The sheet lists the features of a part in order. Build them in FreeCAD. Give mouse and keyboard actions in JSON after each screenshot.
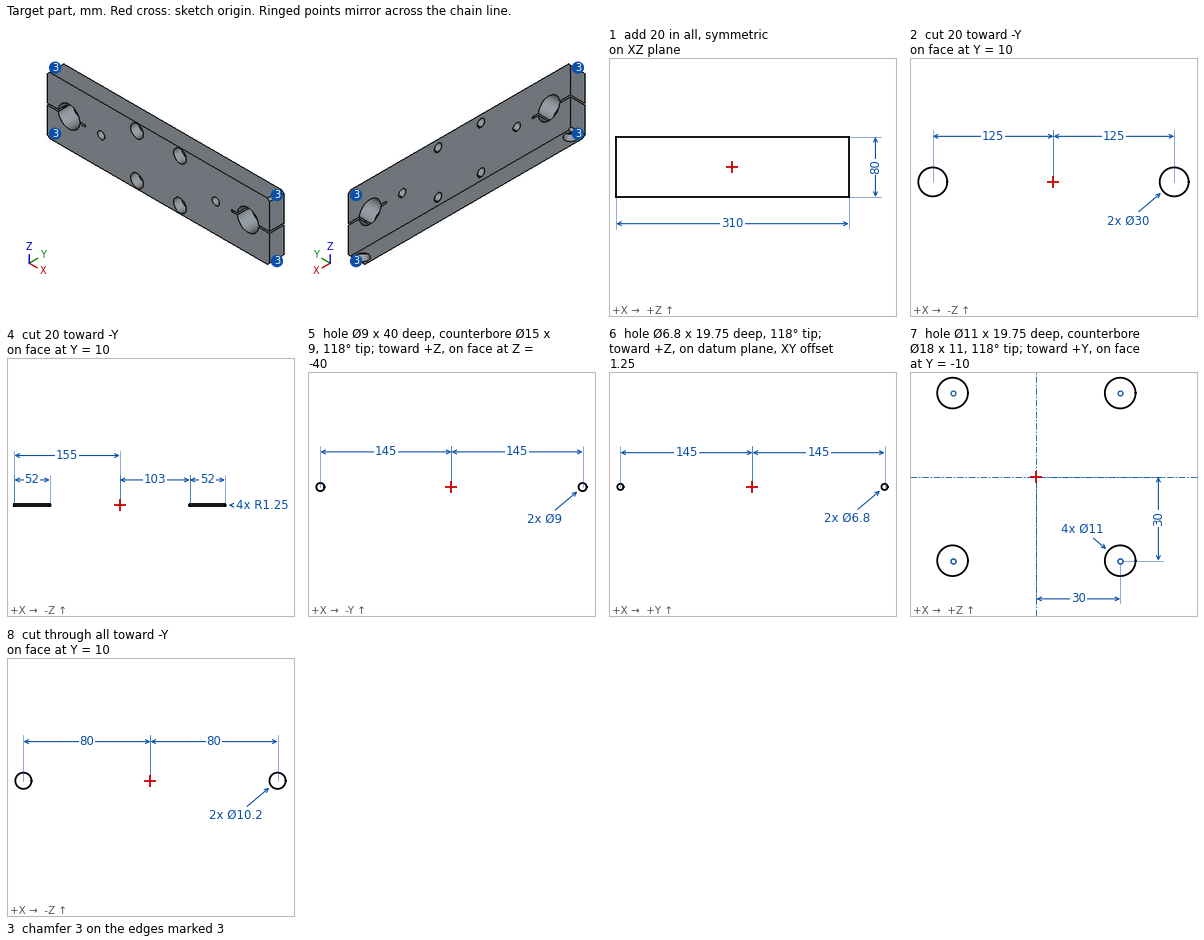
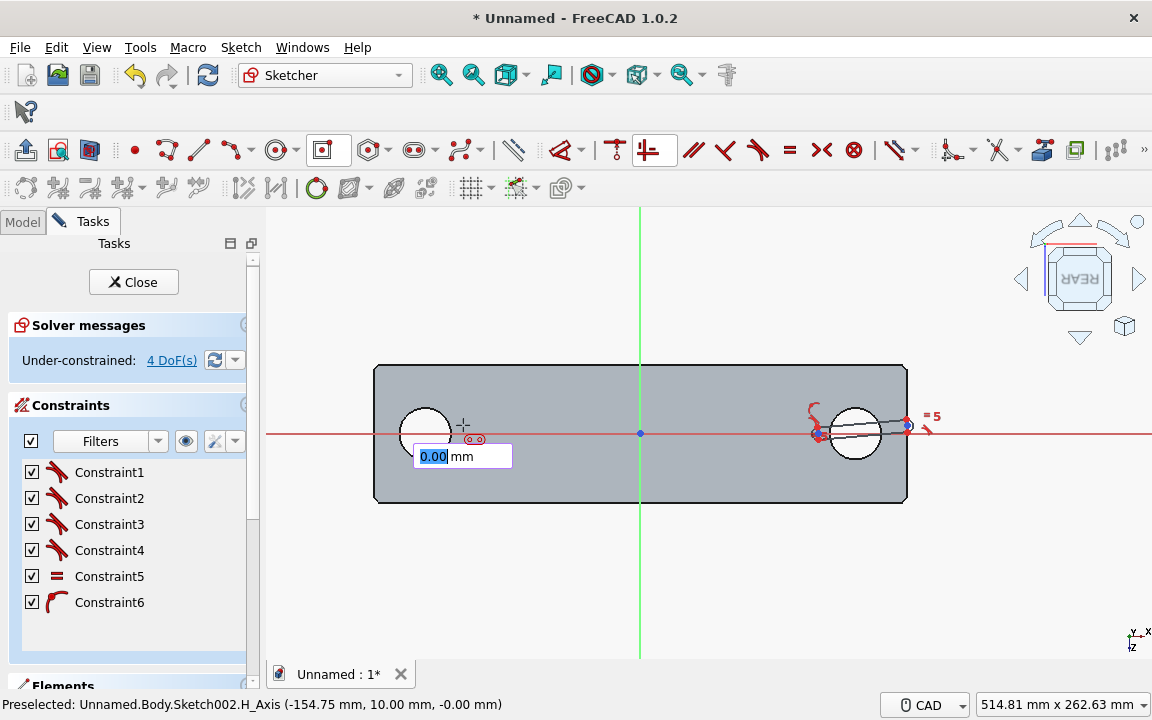
{"action": "scroll", "coordinate": [418, 436], "scroll_direction": "up", "scroll_amount": 10}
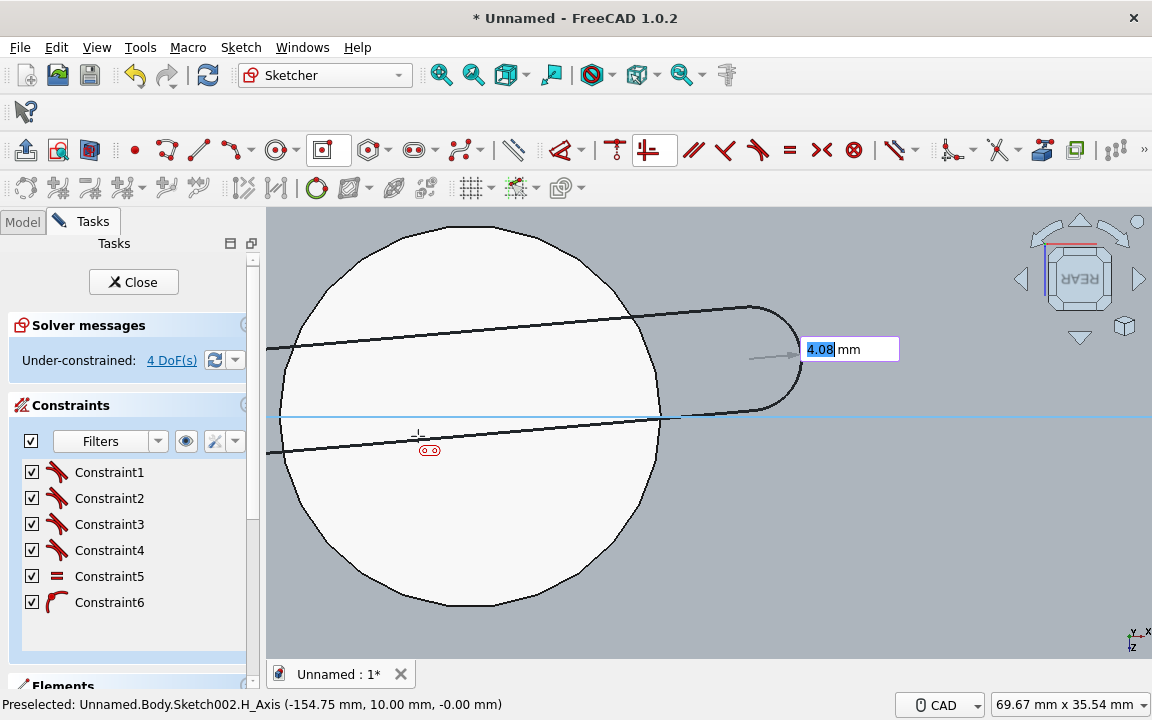
{"action": "left_click", "coordinate": [419, 432]}
{"action": "key", "text": "Escape"}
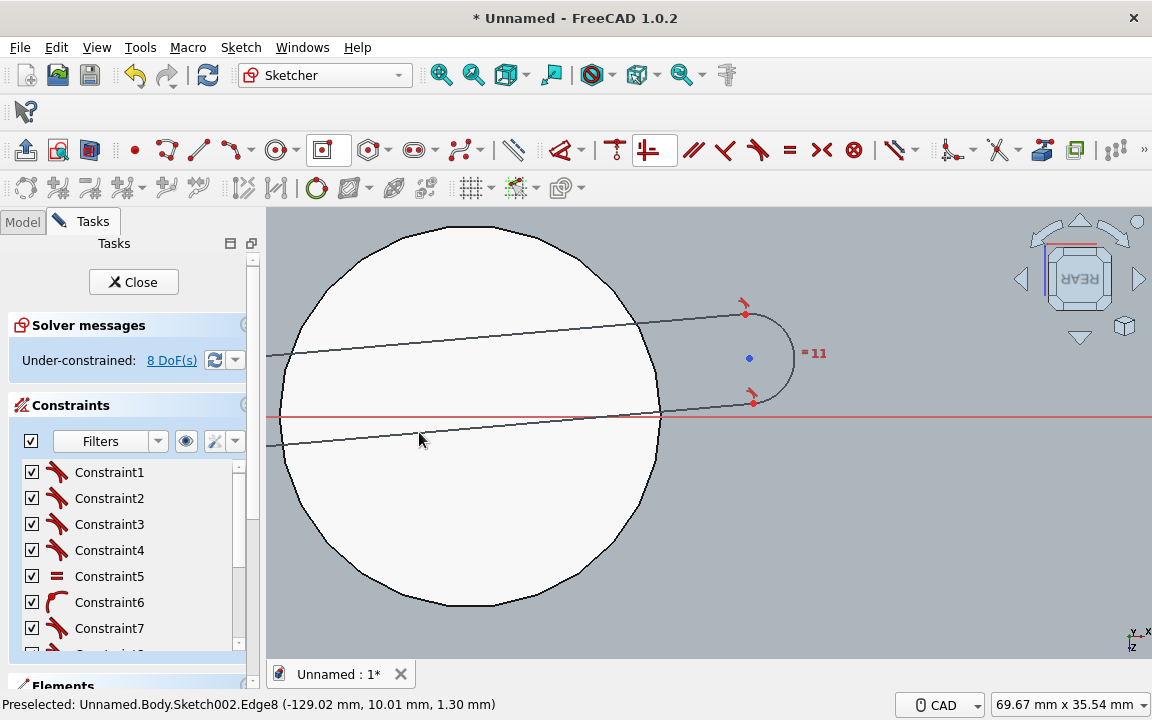
{"action": "scroll", "coordinate": [418, 436], "scroll_direction": "down", "scroll_amount": 10}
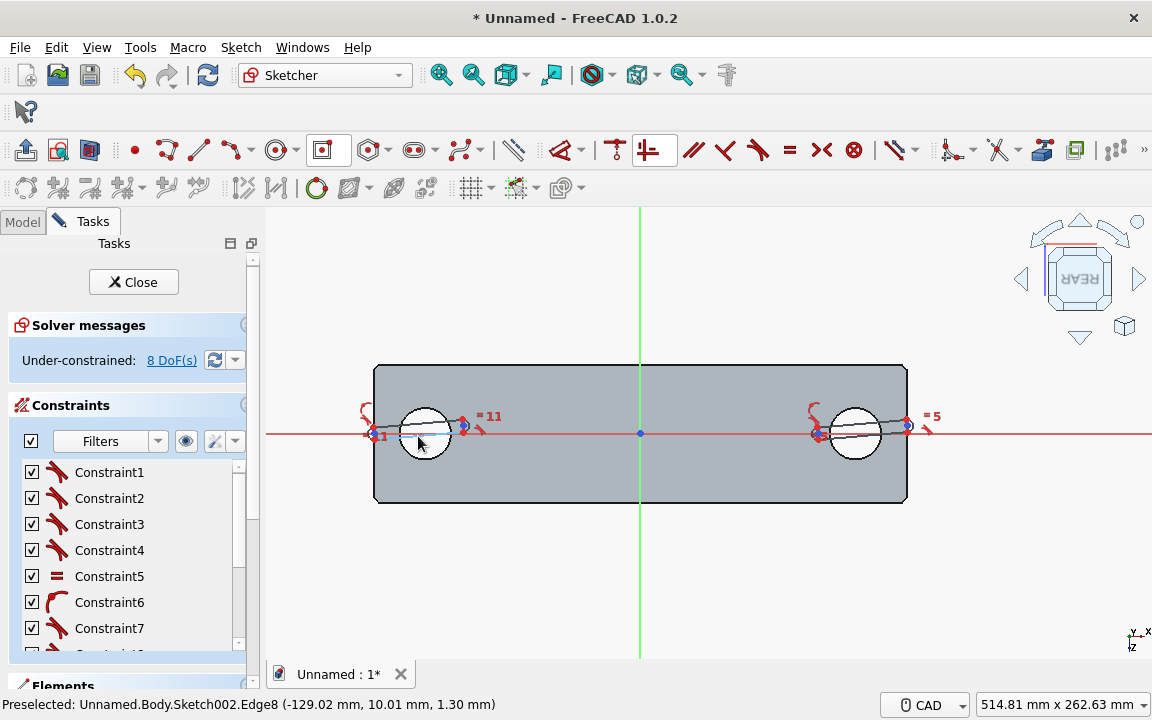
{"action": "scroll", "coordinate": [844, 425], "scroll_direction": "up", "scroll_amount": 3}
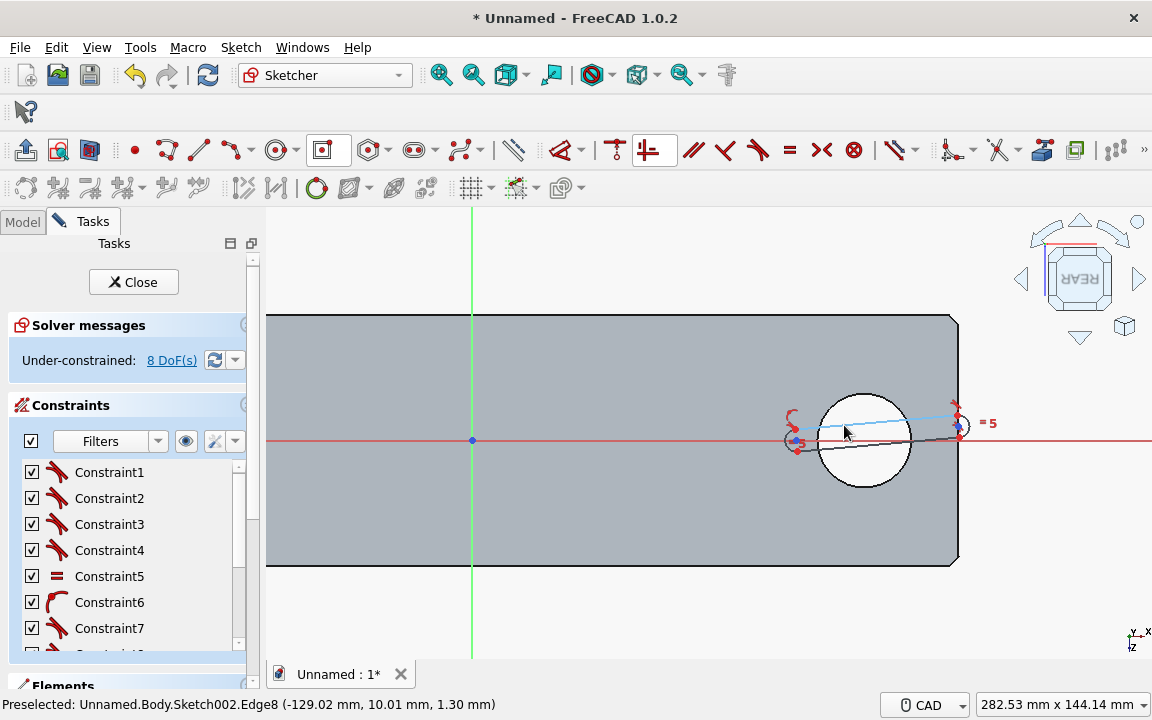
{"action": "left_click", "coordinate": [844, 425]}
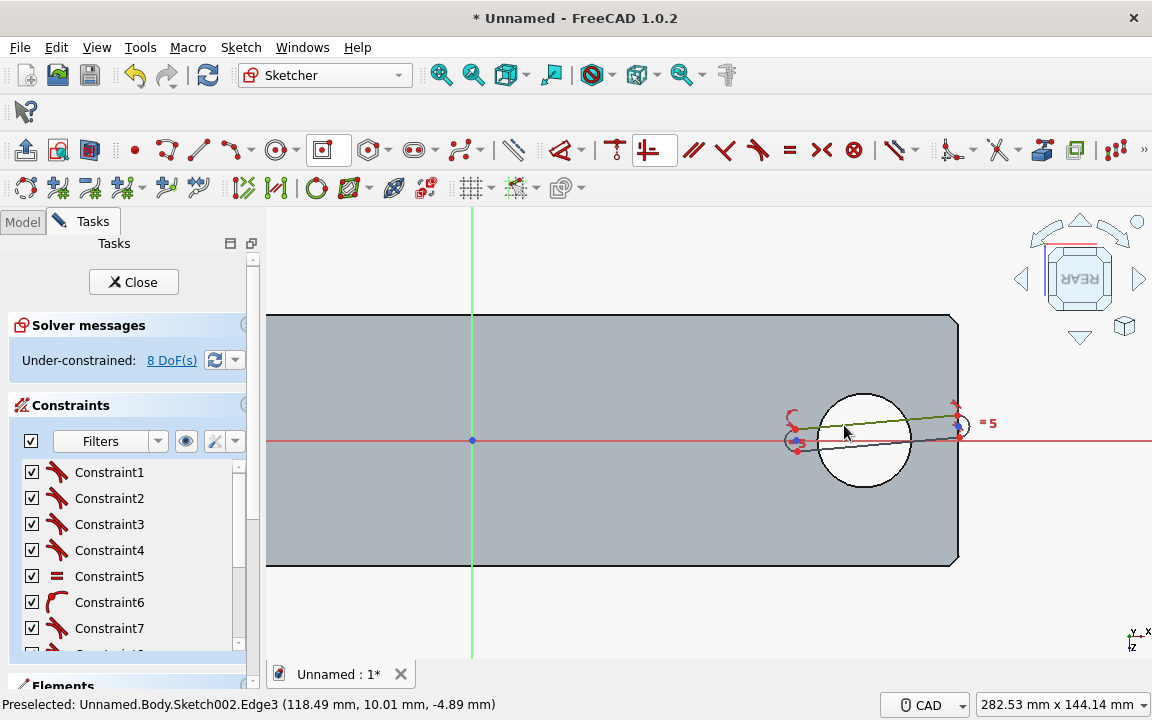
{"action": "key", "text": "h"}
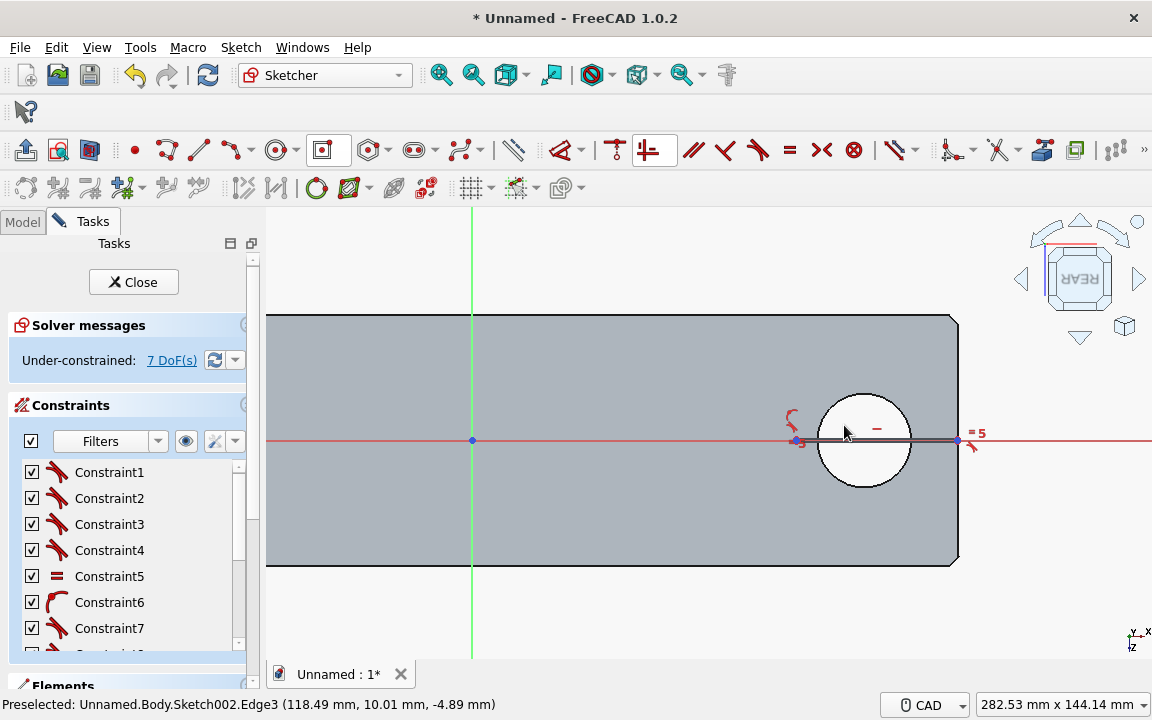
{"action": "scroll", "coordinate": [845, 424], "scroll_direction": "down", "scroll_amount": 3}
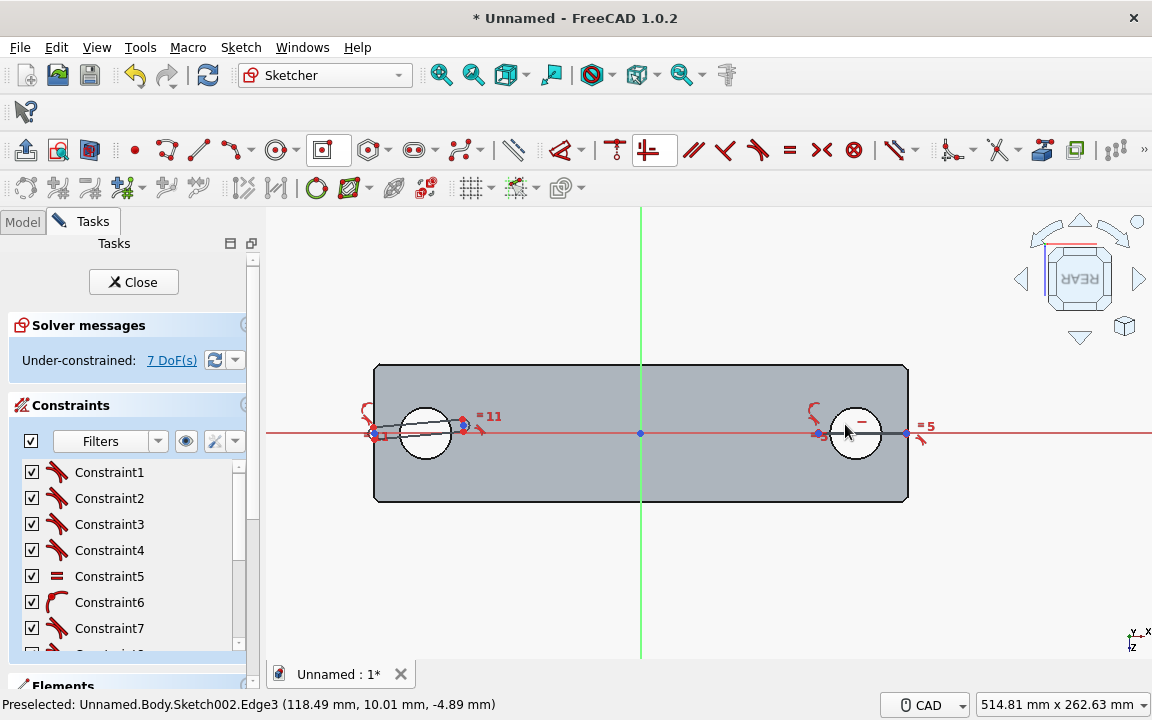
{"action": "scroll", "coordinate": [401, 425], "scroll_direction": "up", "scroll_amount": 3}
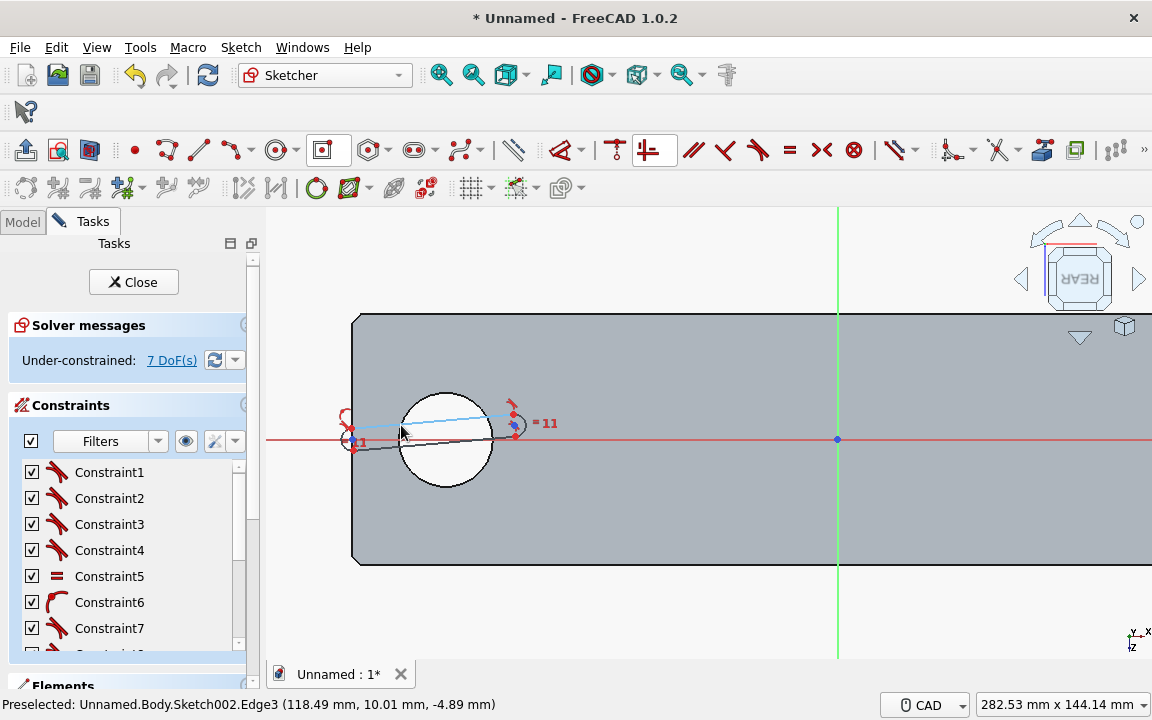
{"action": "left_click", "coordinate": [400, 424]}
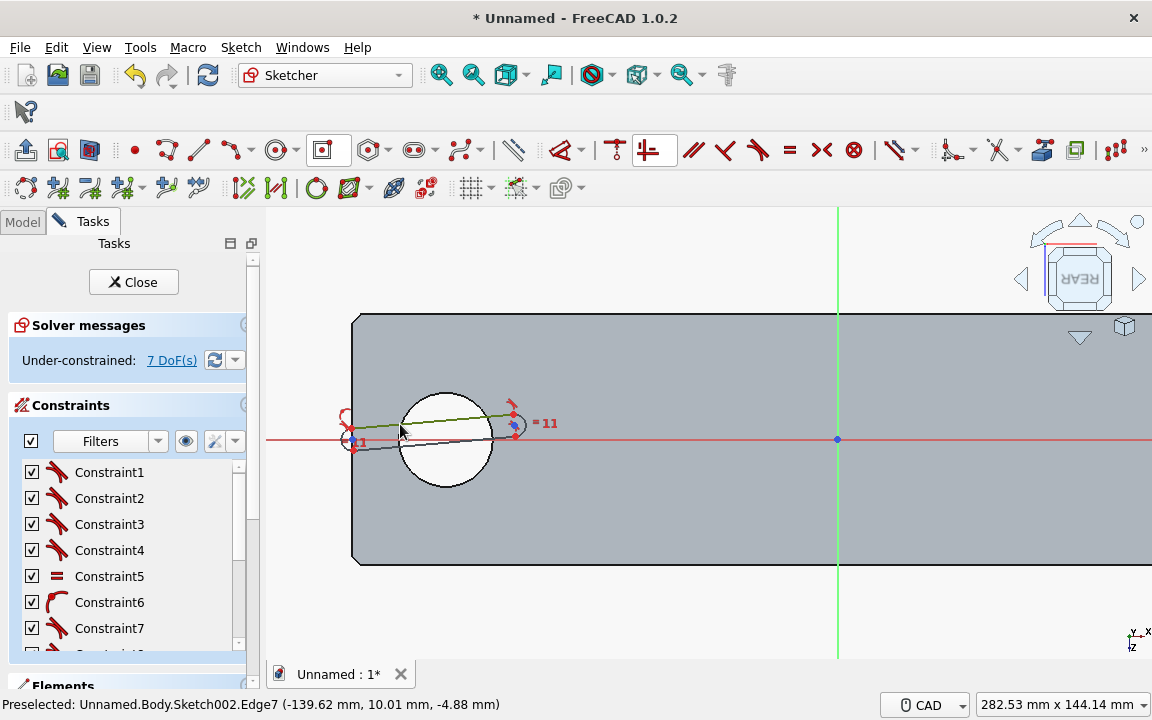
{"action": "key", "text": "h"}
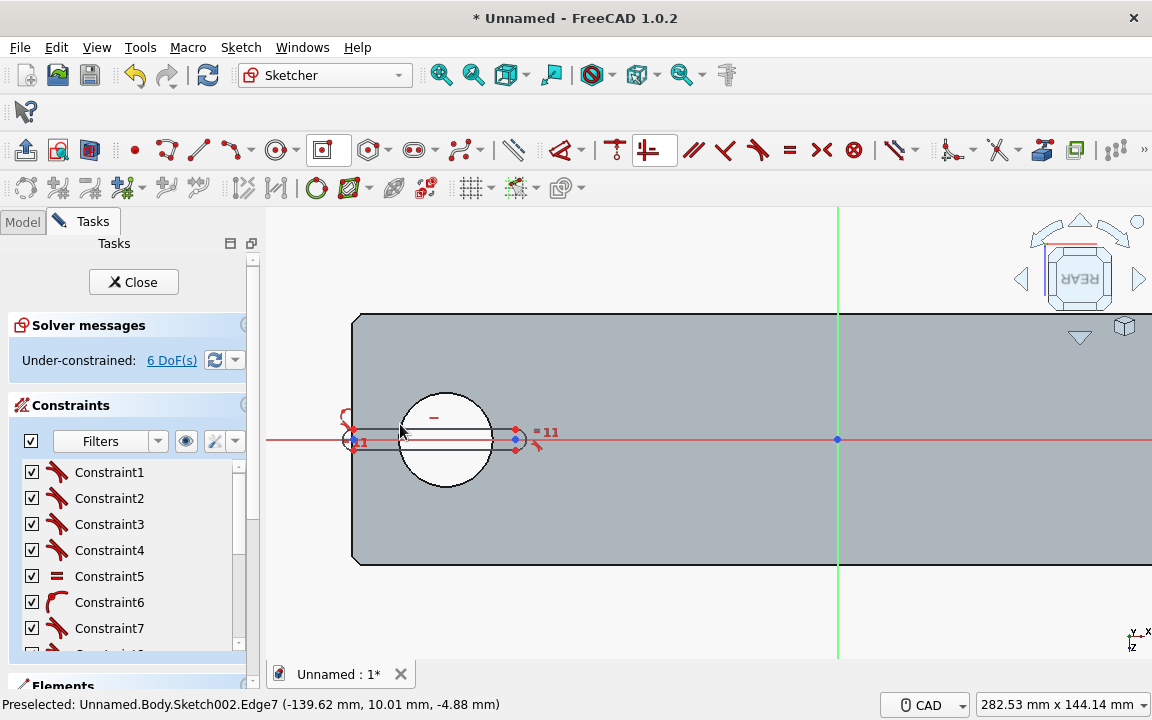
{"action": "scroll", "coordinate": [401, 425], "scroll_direction": "down", "scroll_amount": 3}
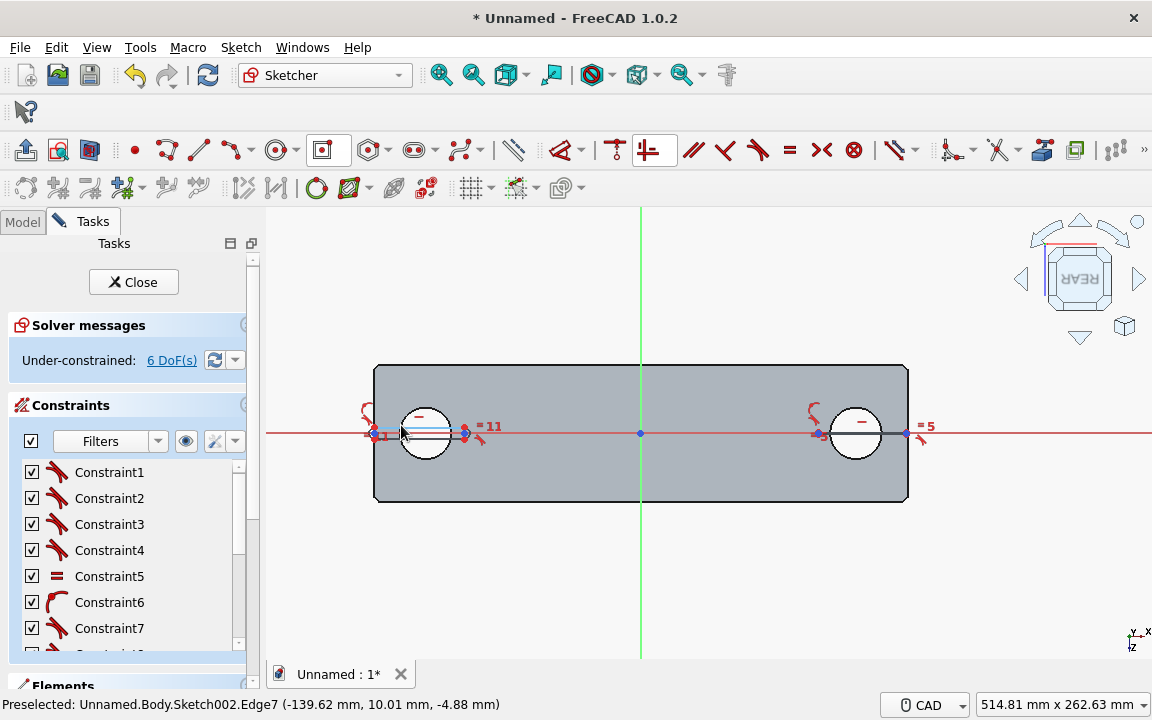
{"action": "scroll", "coordinate": [818, 433], "scroll_direction": "up", "scroll_amount": 13}